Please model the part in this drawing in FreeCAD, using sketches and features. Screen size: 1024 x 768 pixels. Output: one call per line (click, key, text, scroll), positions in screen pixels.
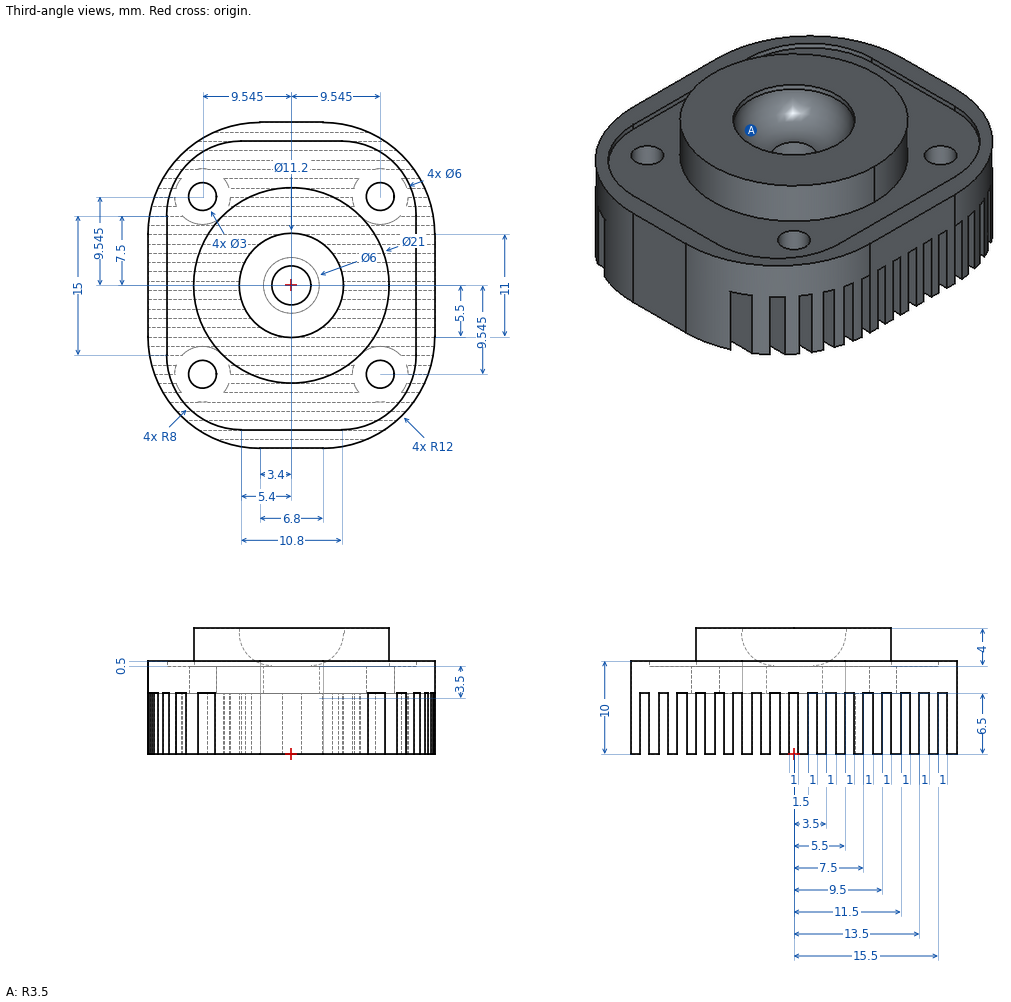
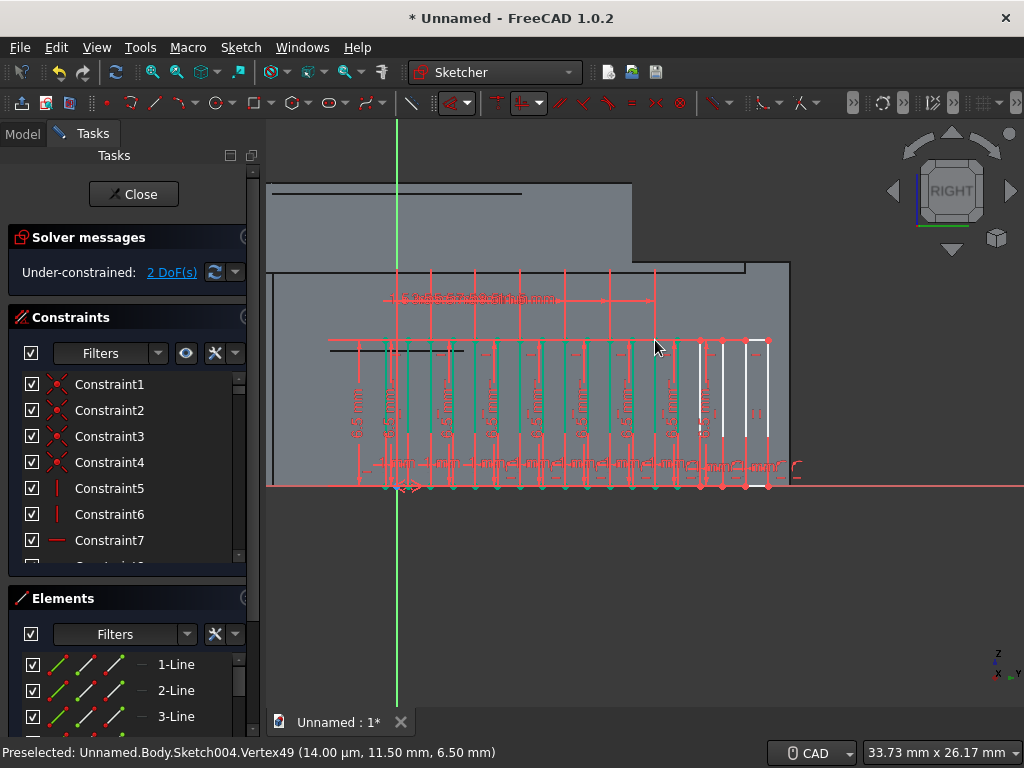
click(700, 340)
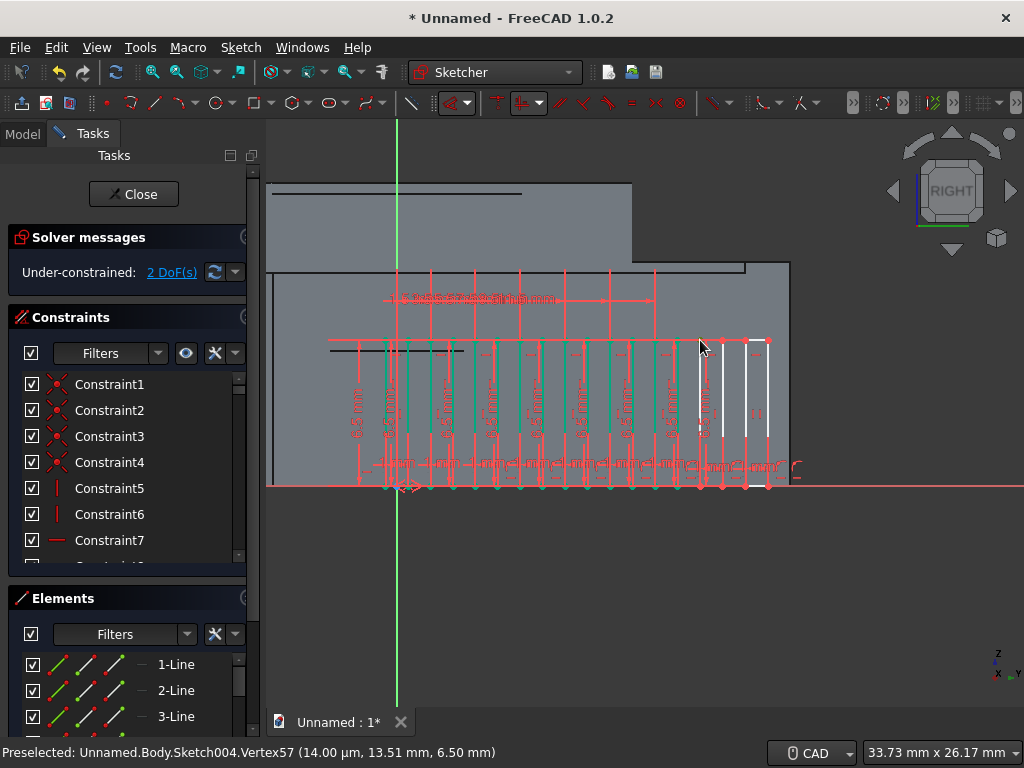
key(l)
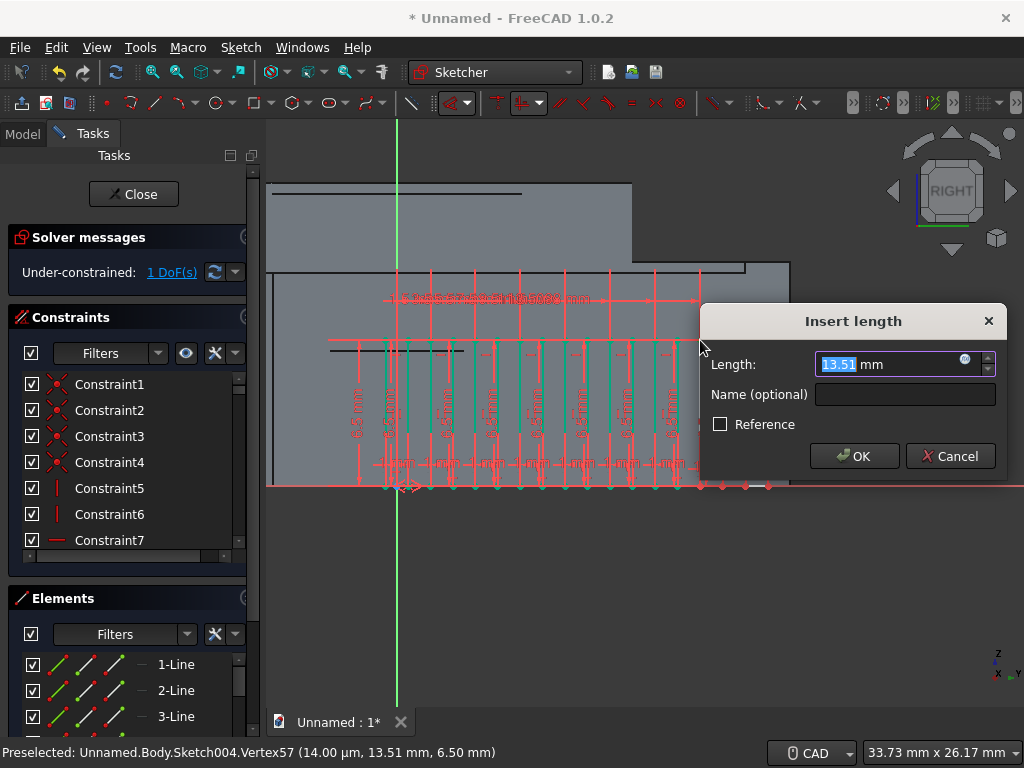
text(13.5)
key(Return)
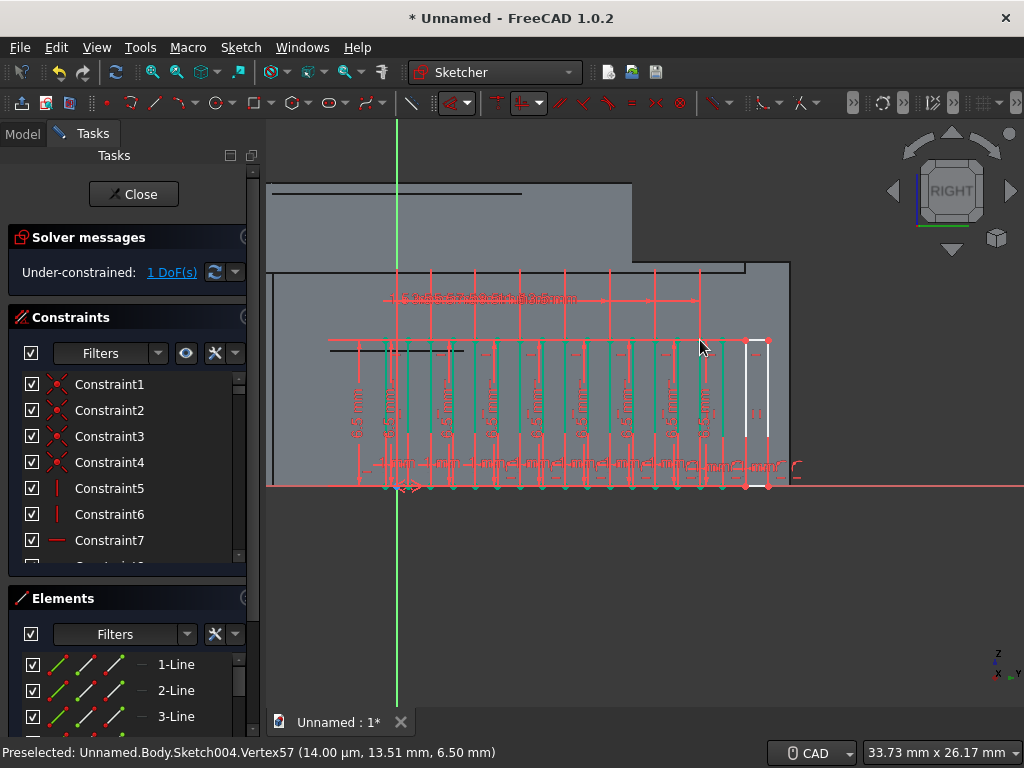
click(746, 340)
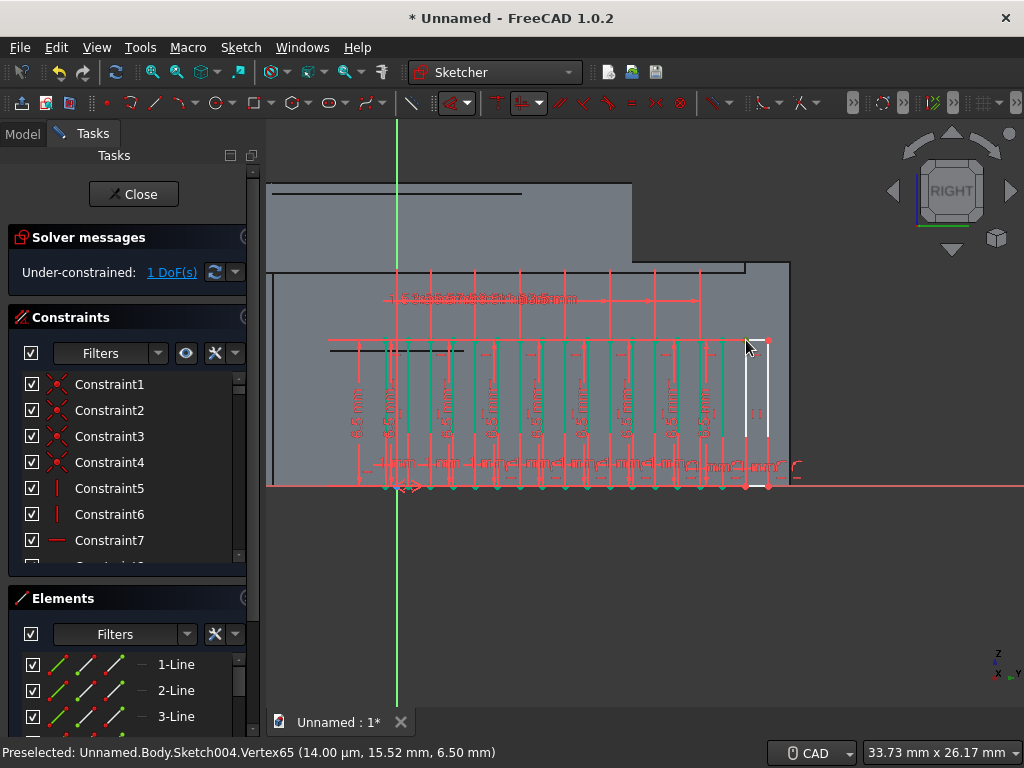
key(l)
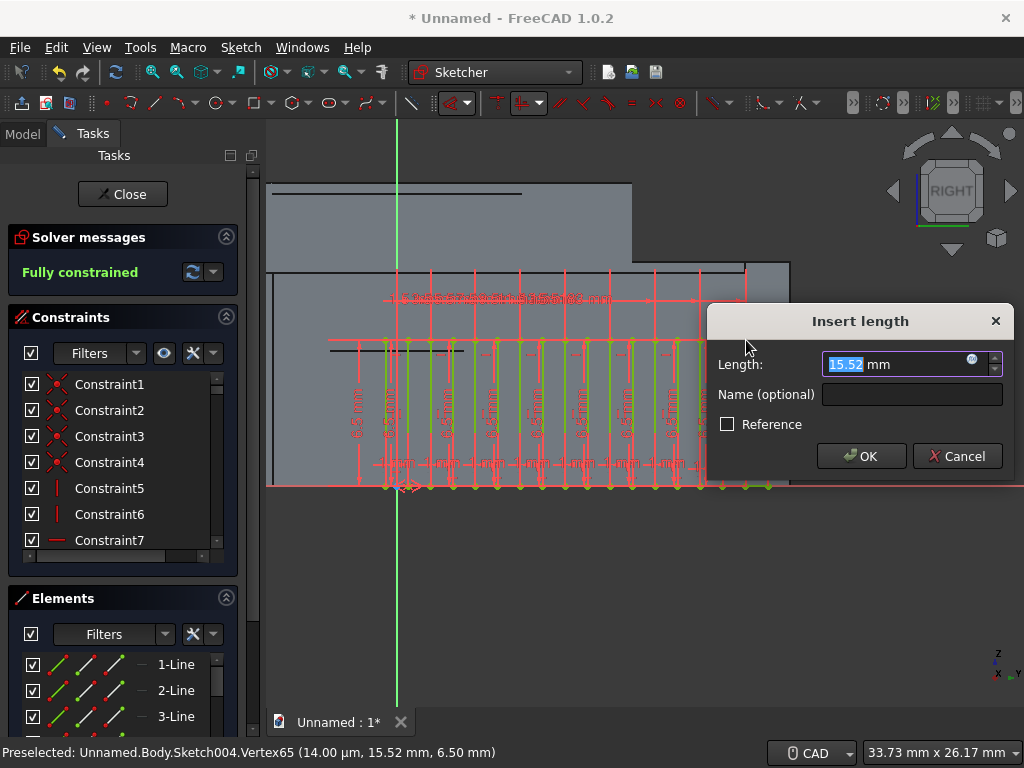
text(15.5)
key(Return)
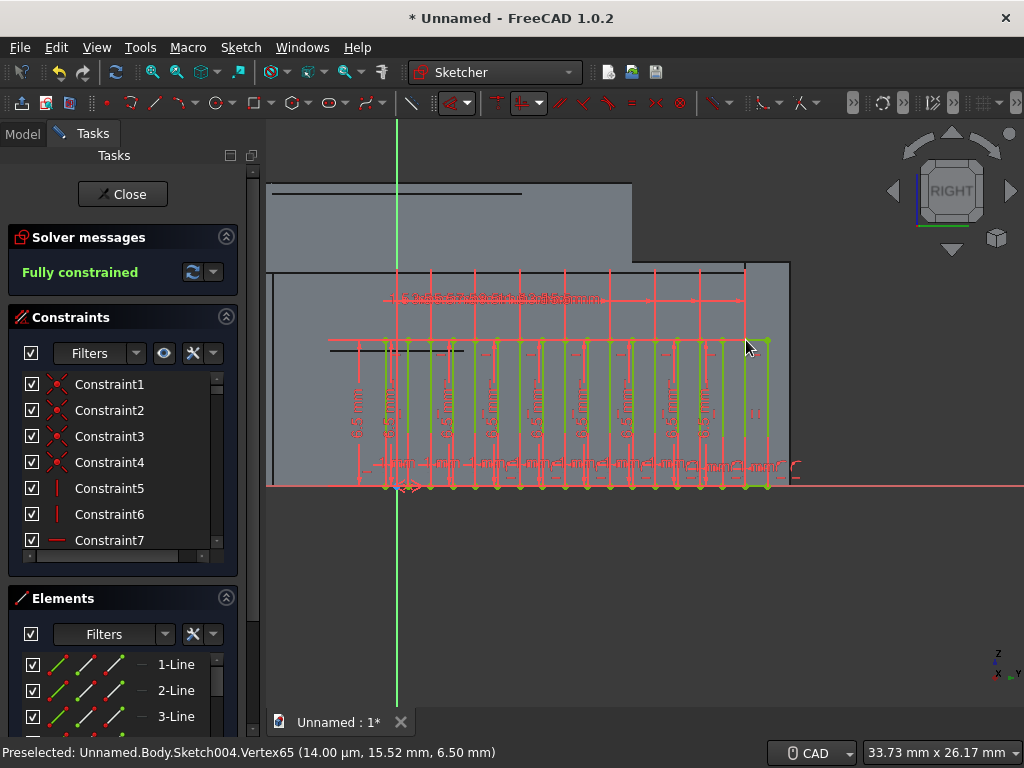
click(123, 194)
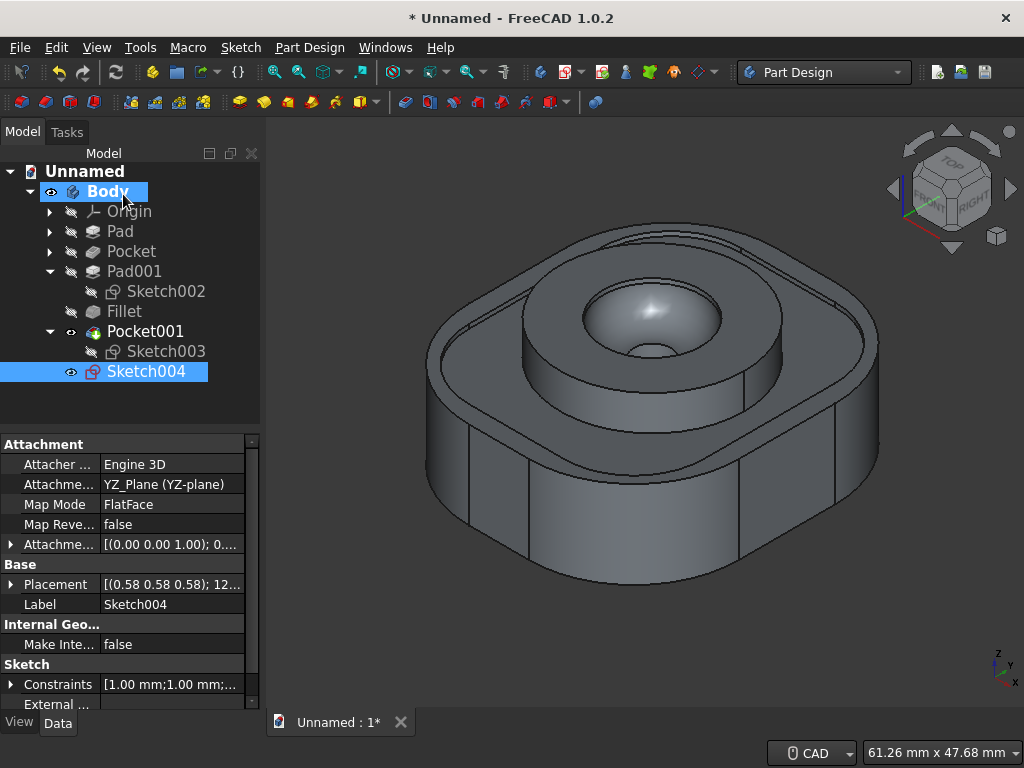
click(406, 102)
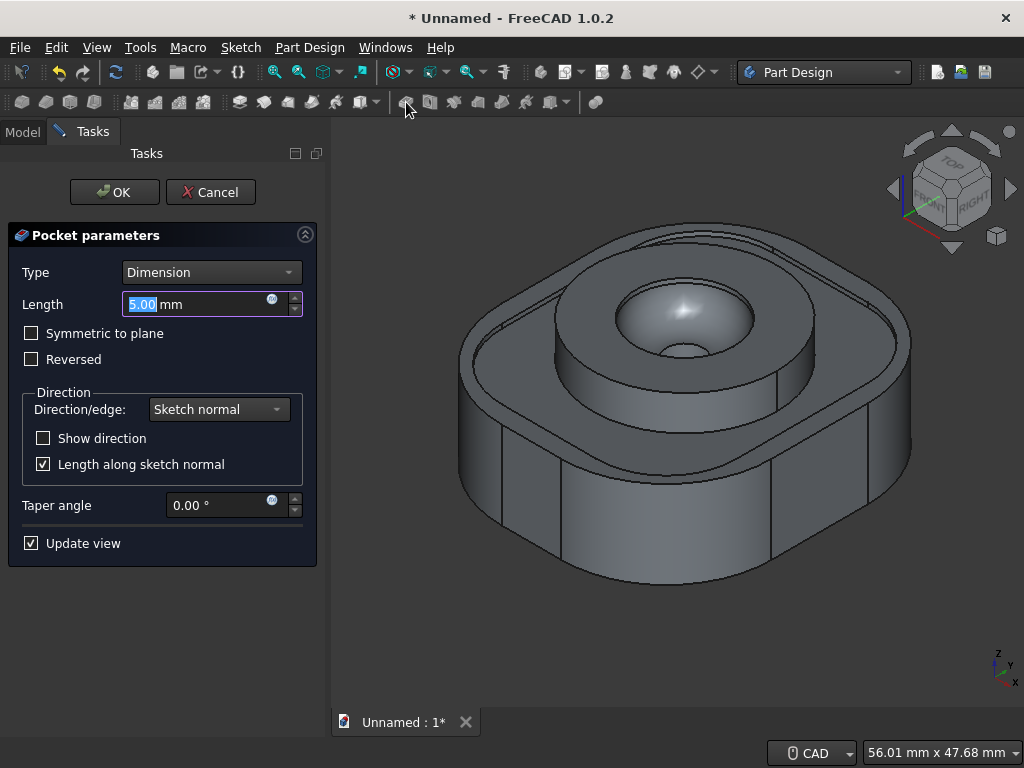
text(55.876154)
key(Tab)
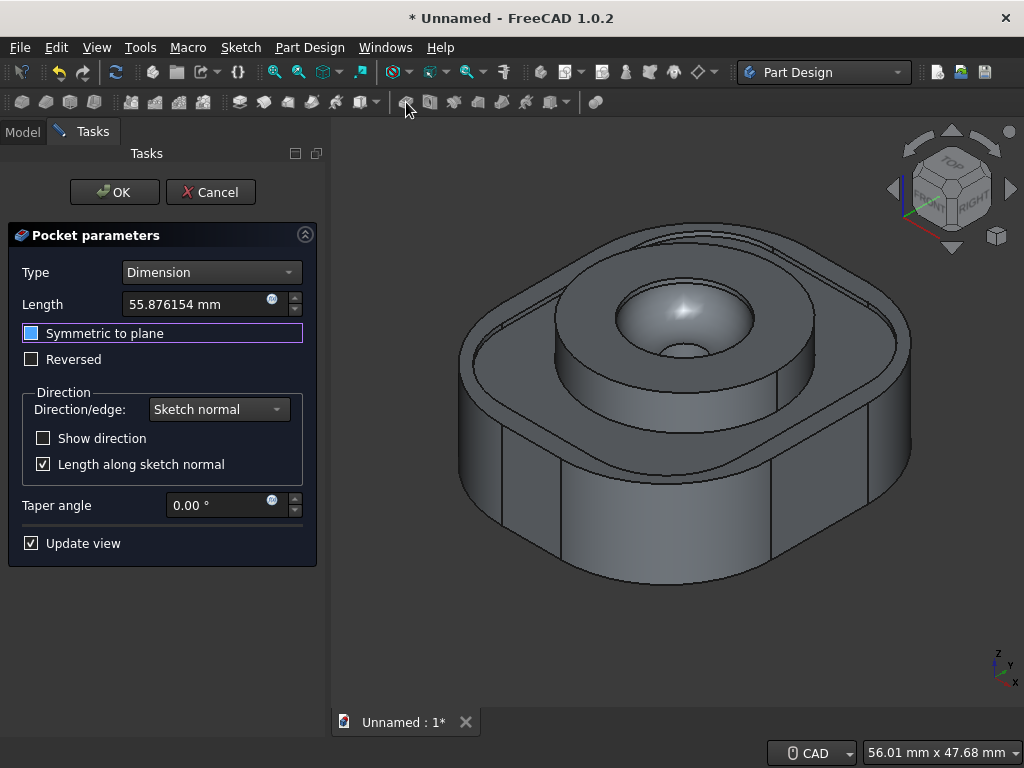
click(30, 333)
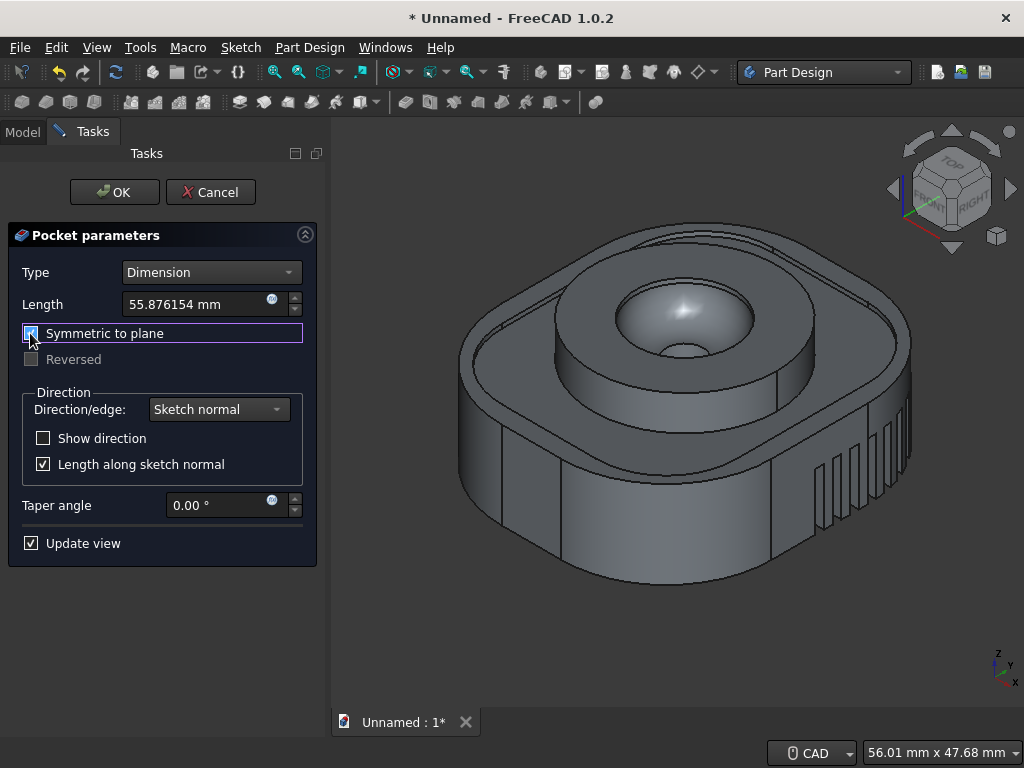
click(115, 192)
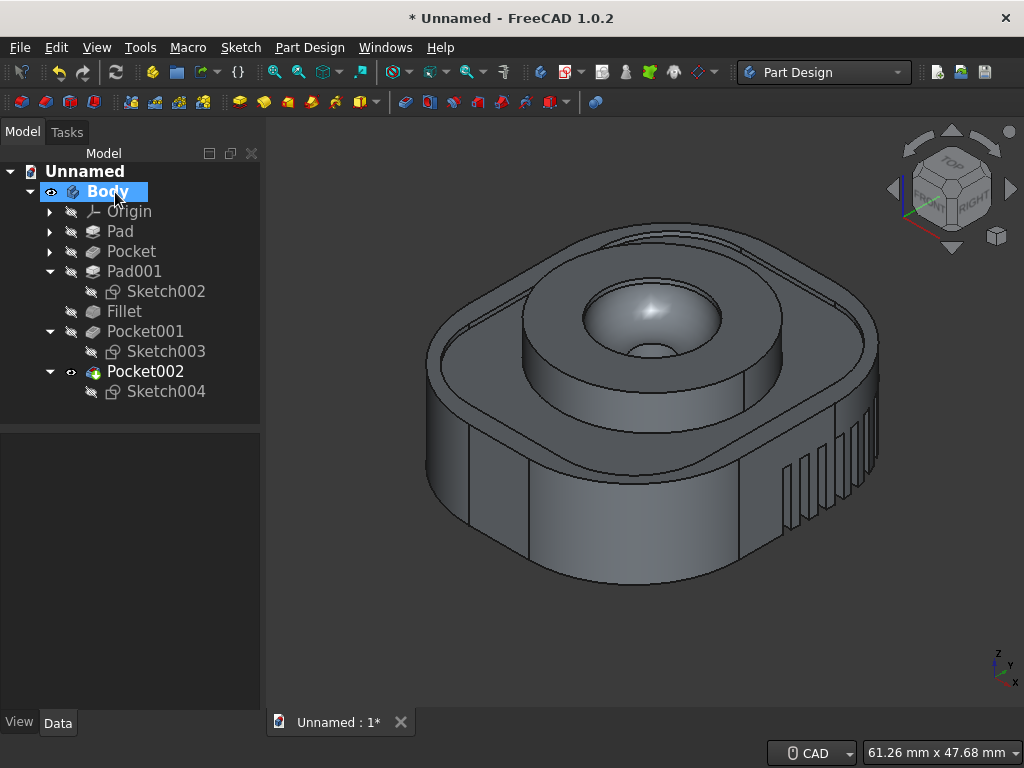
click(116, 372)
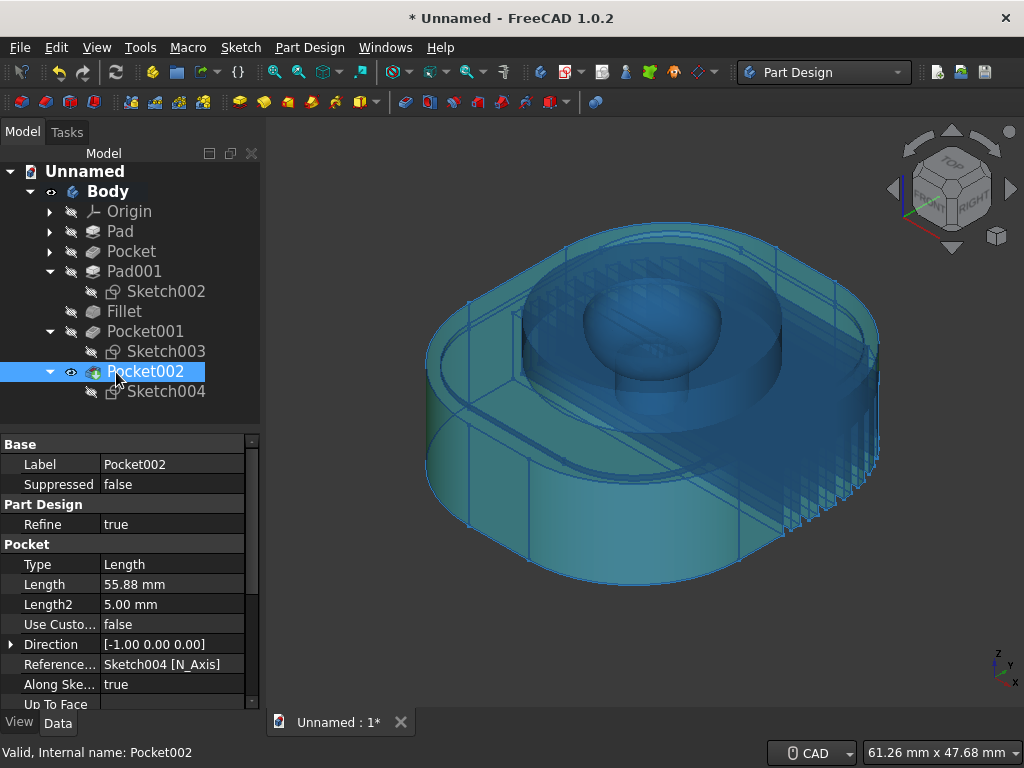
click(132, 102)